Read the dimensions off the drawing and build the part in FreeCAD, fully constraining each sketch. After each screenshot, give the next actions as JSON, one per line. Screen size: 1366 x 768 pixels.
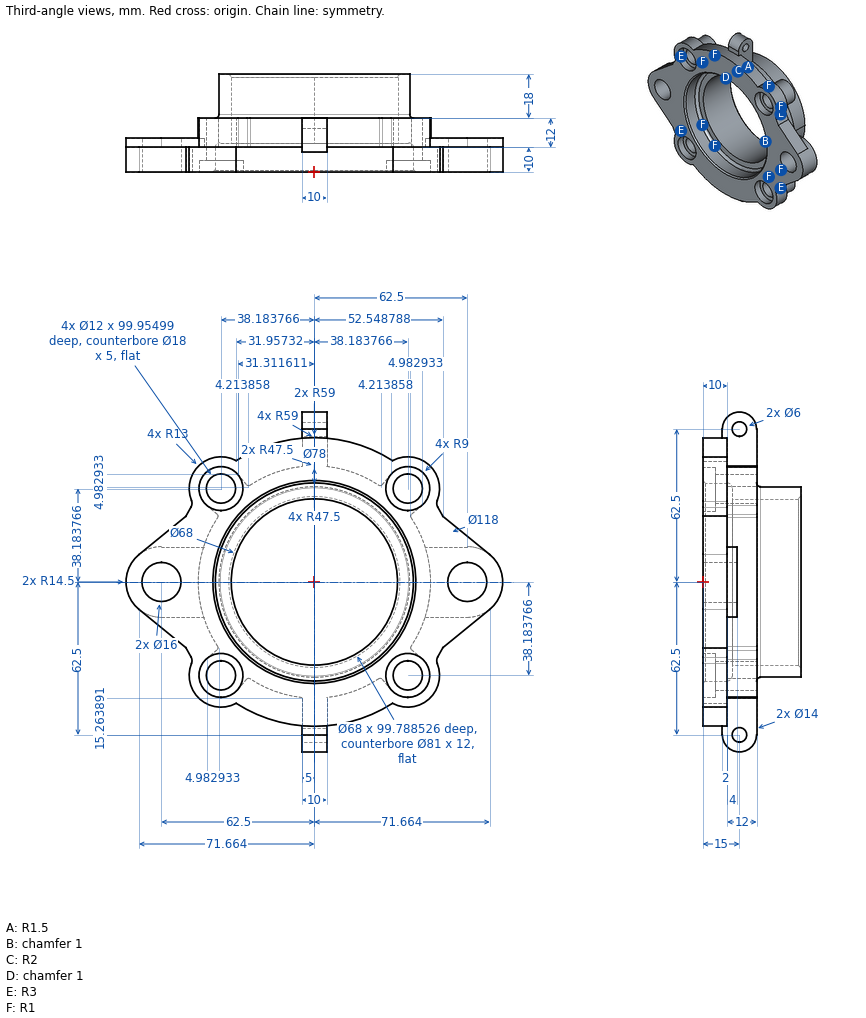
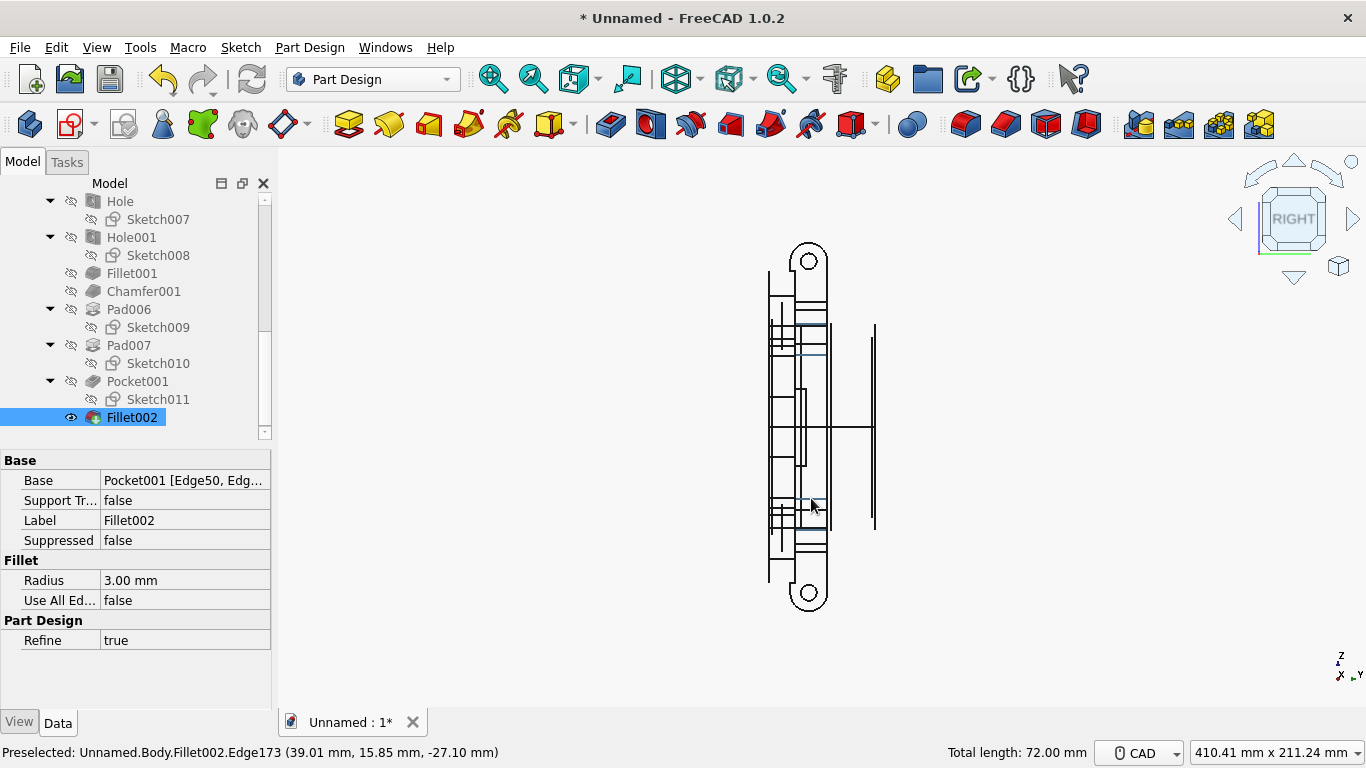
{"action": "key", "text": "5"}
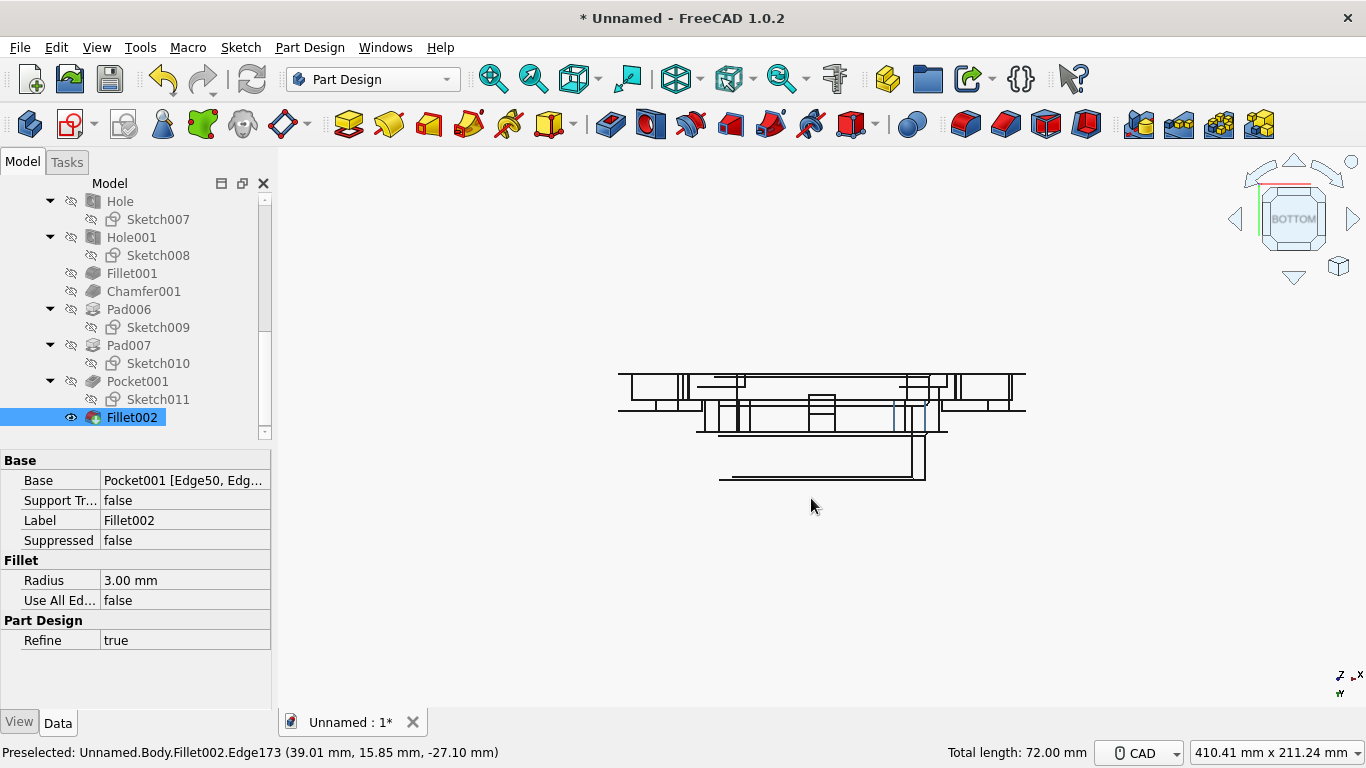
{"action": "left_click", "coordinate": [494, 80]}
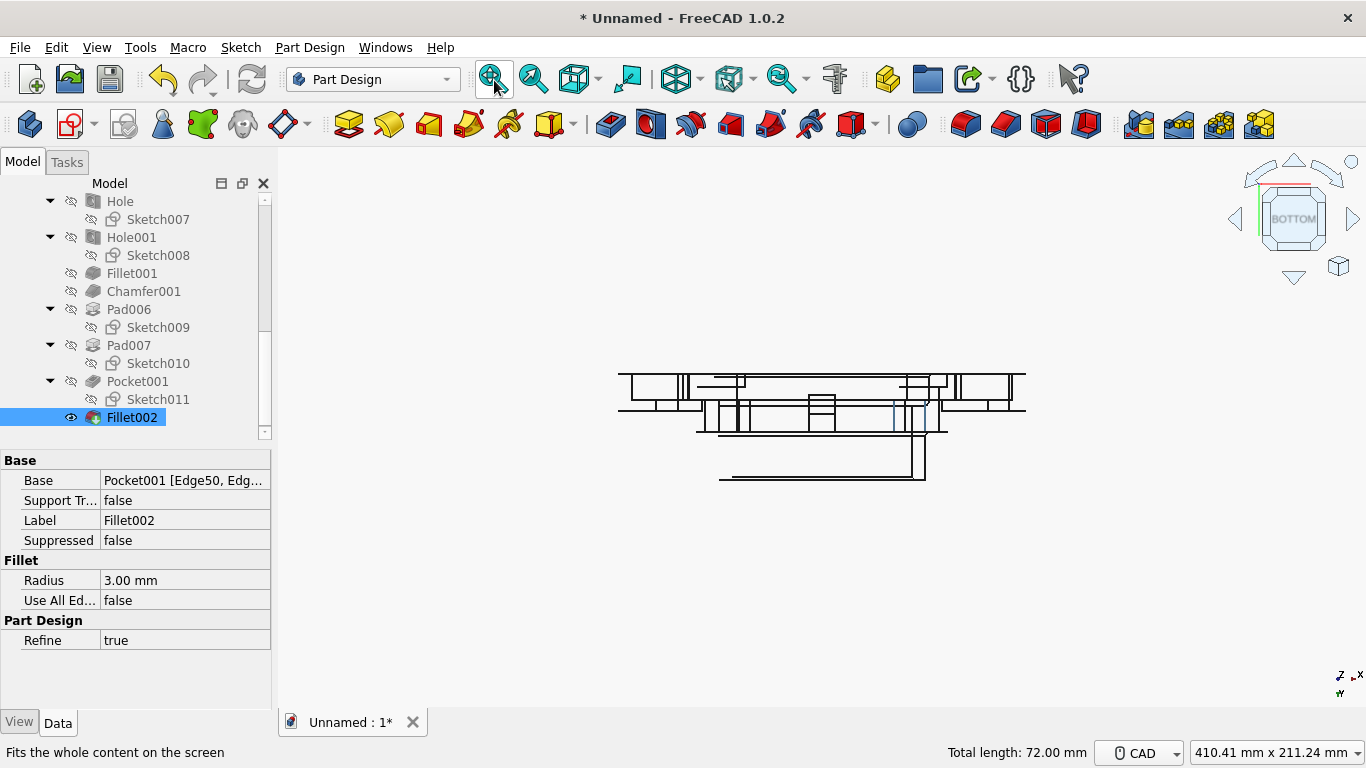
{"action": "left_click", "coordinate": [750, 415], "text": "ctrl"}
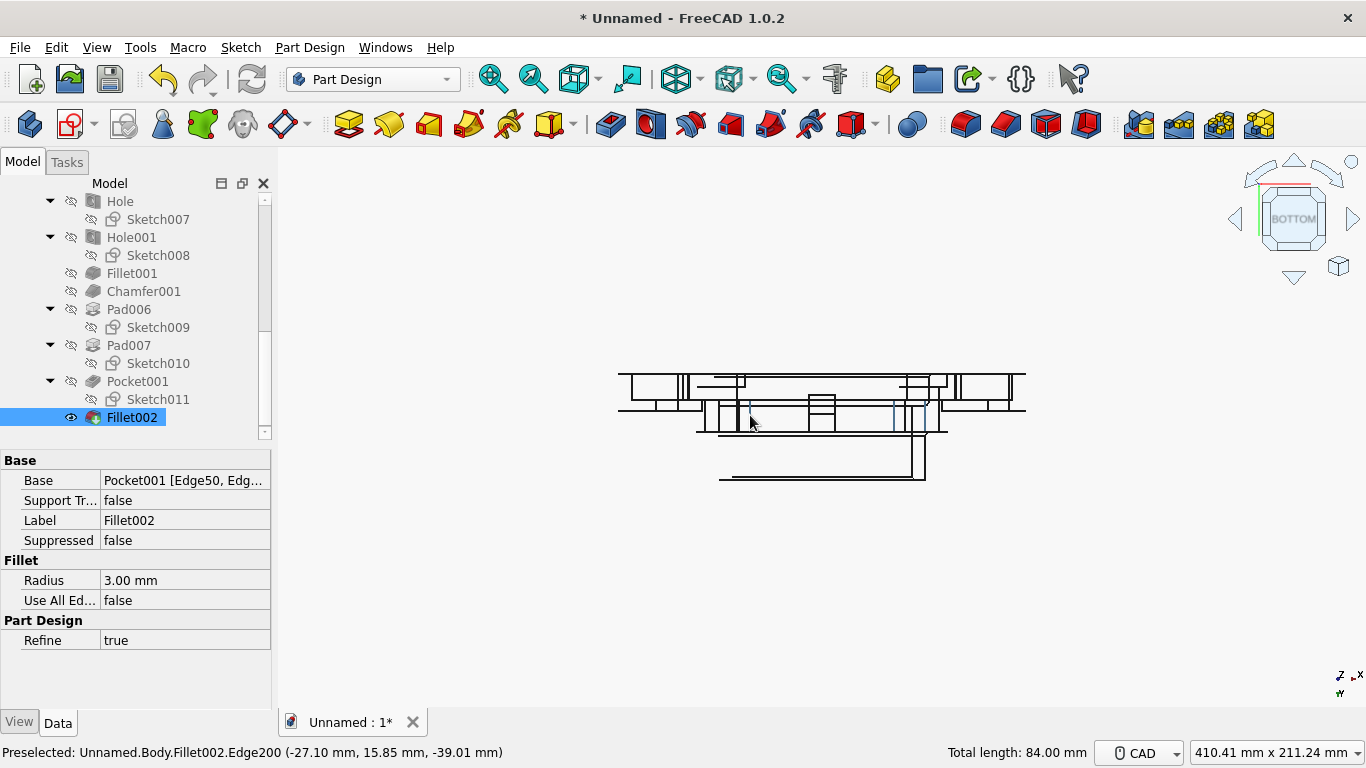
{"action": "left_click", "coordinate": [719, 415], "text": "ctrl"}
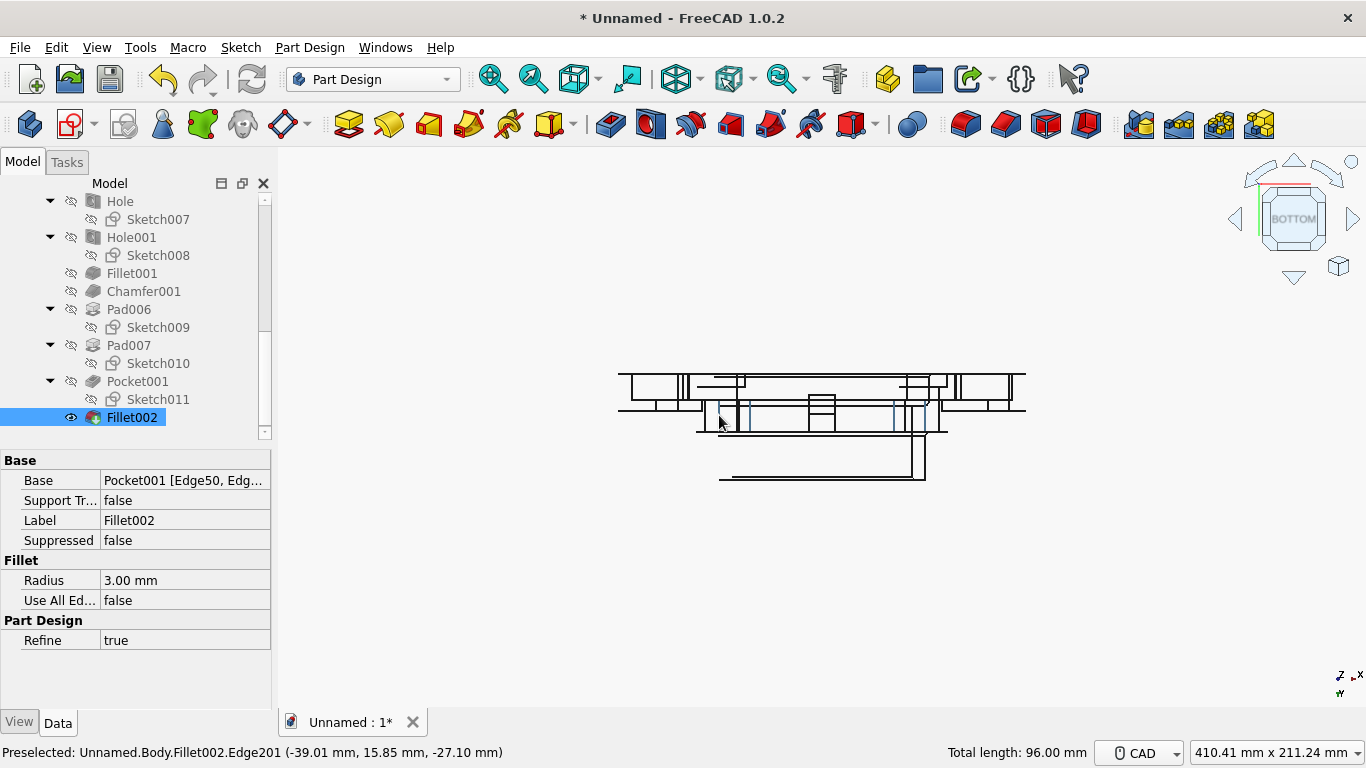
{"action": "key", "text": "v 1"}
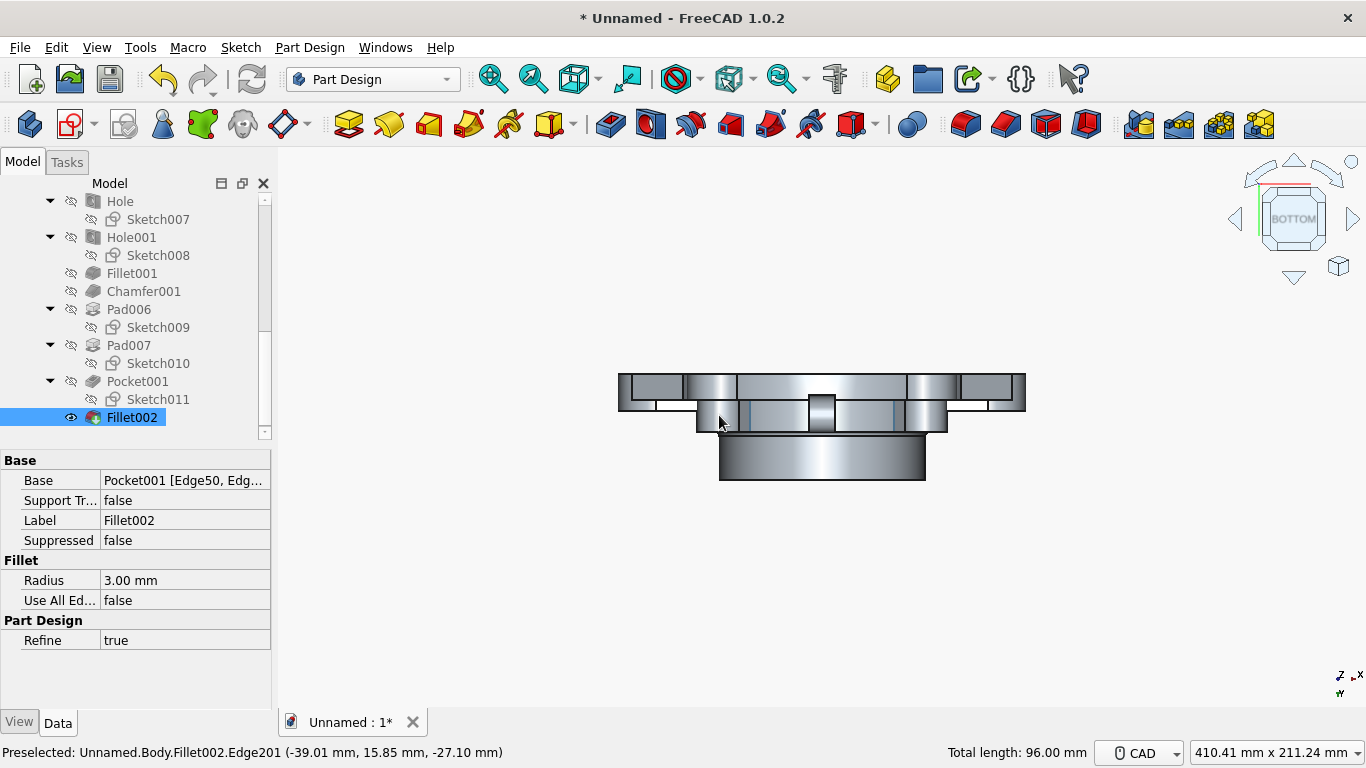
{"action": "left_click", "coordinate": [966, 124]}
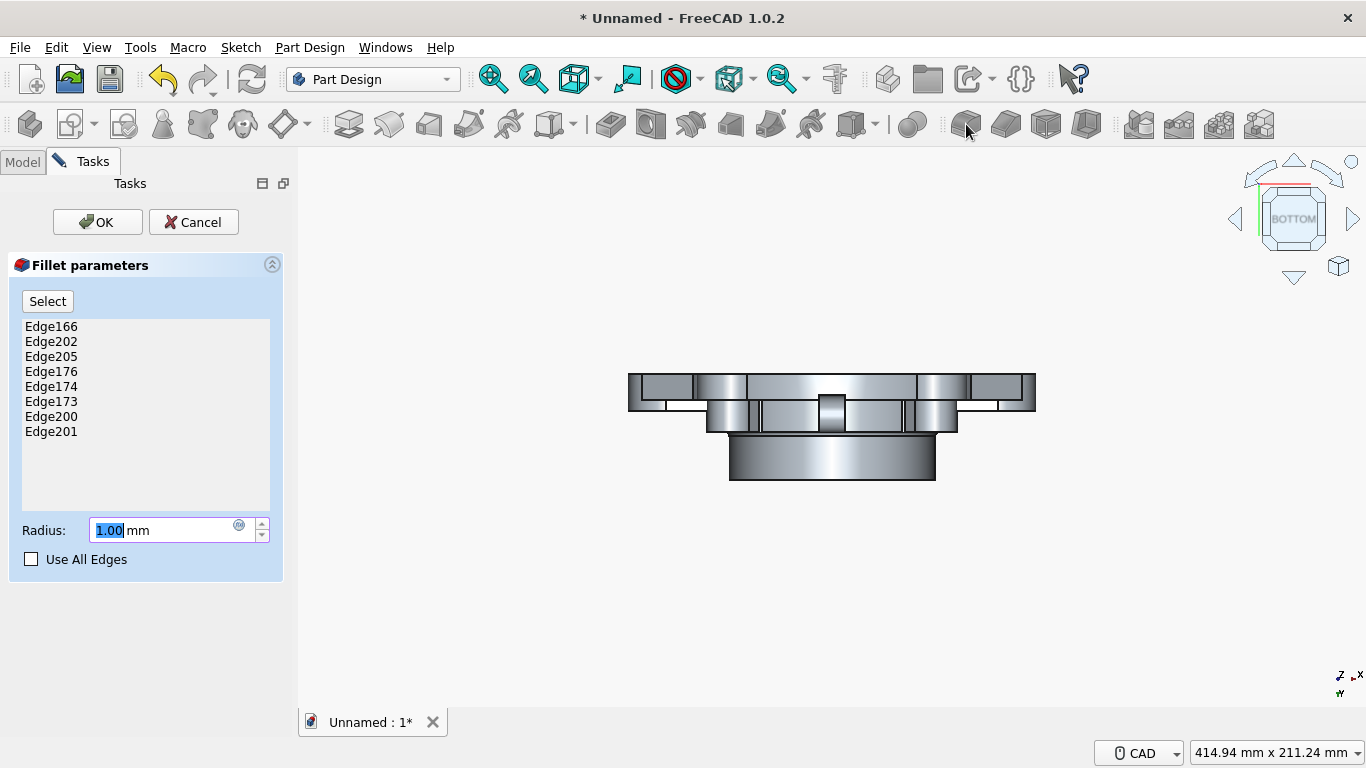
{"action": "type", "text": "1"}
{"action": "key", "text": "Tab"}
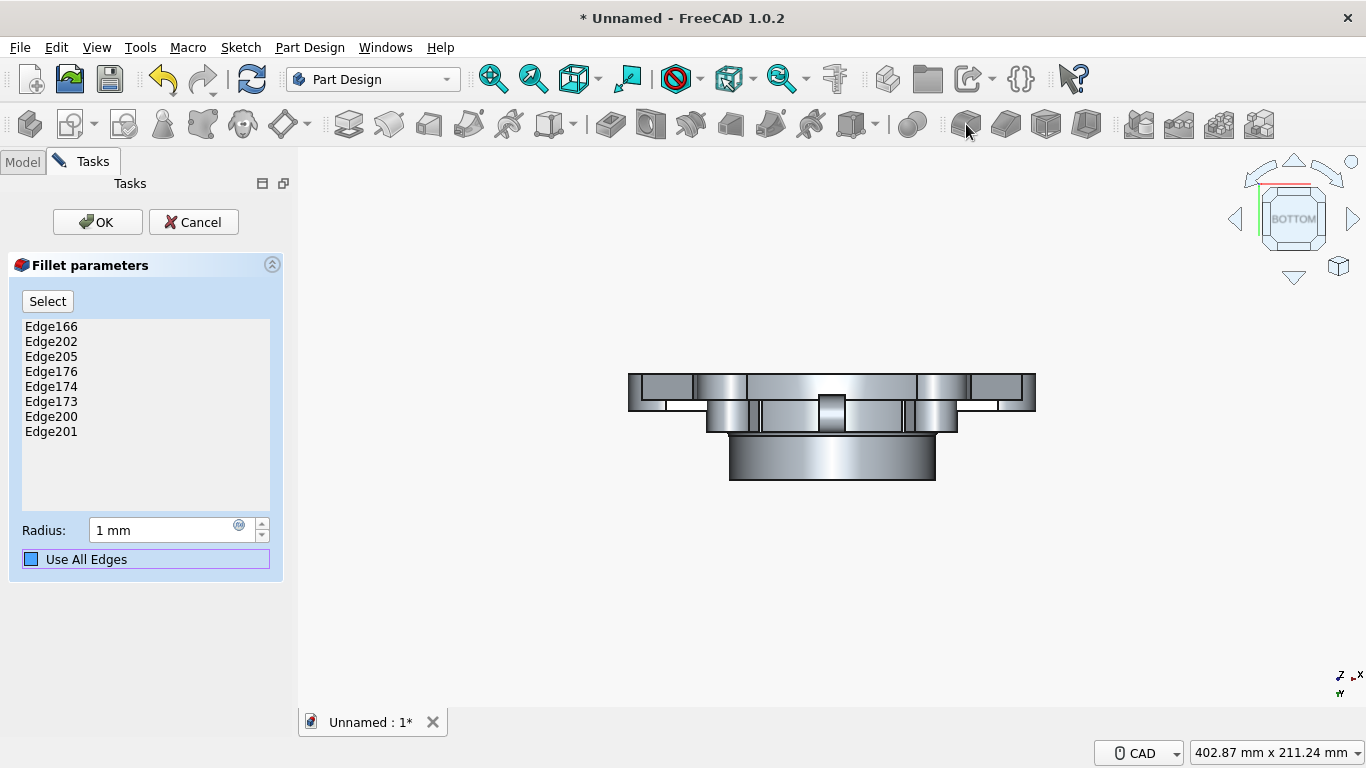
{"action": "left_click", "coordinate": [98, 222]}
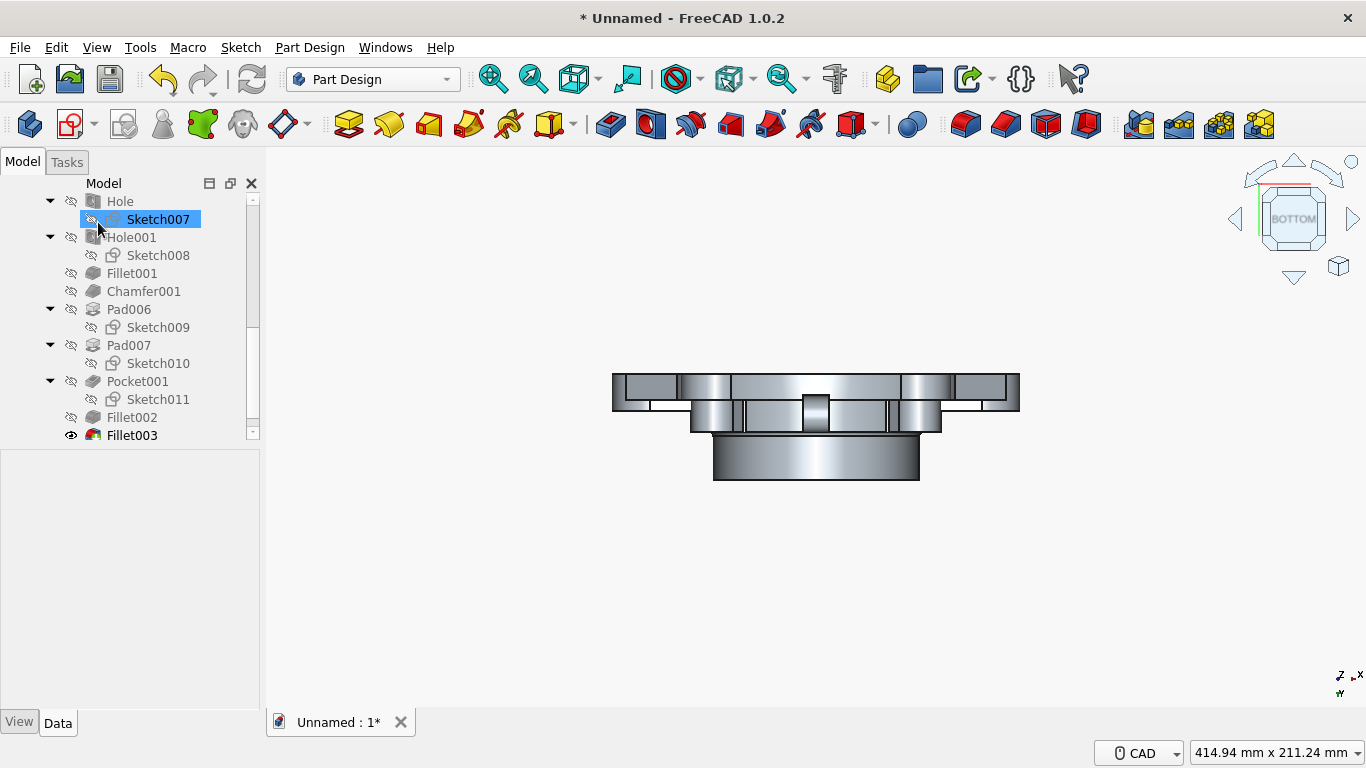
{"action": "key", "text": "0"}